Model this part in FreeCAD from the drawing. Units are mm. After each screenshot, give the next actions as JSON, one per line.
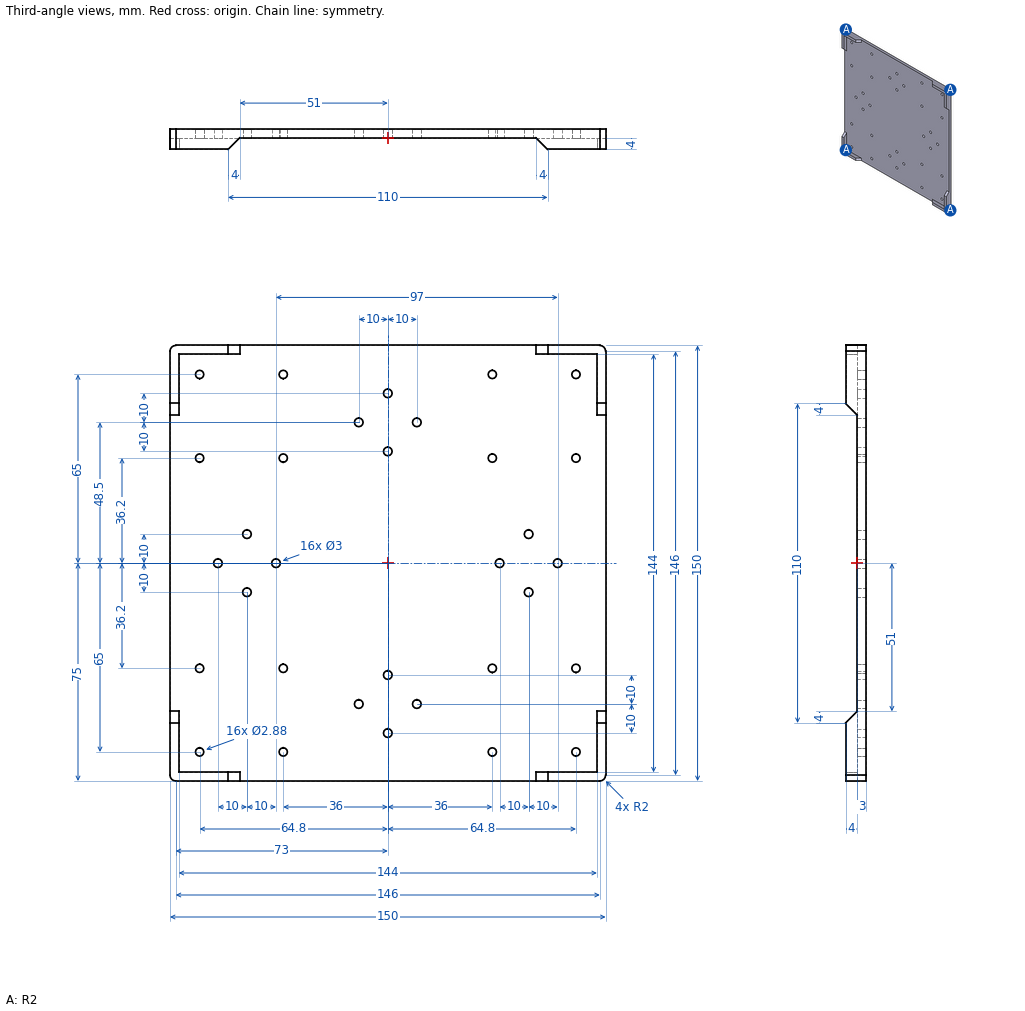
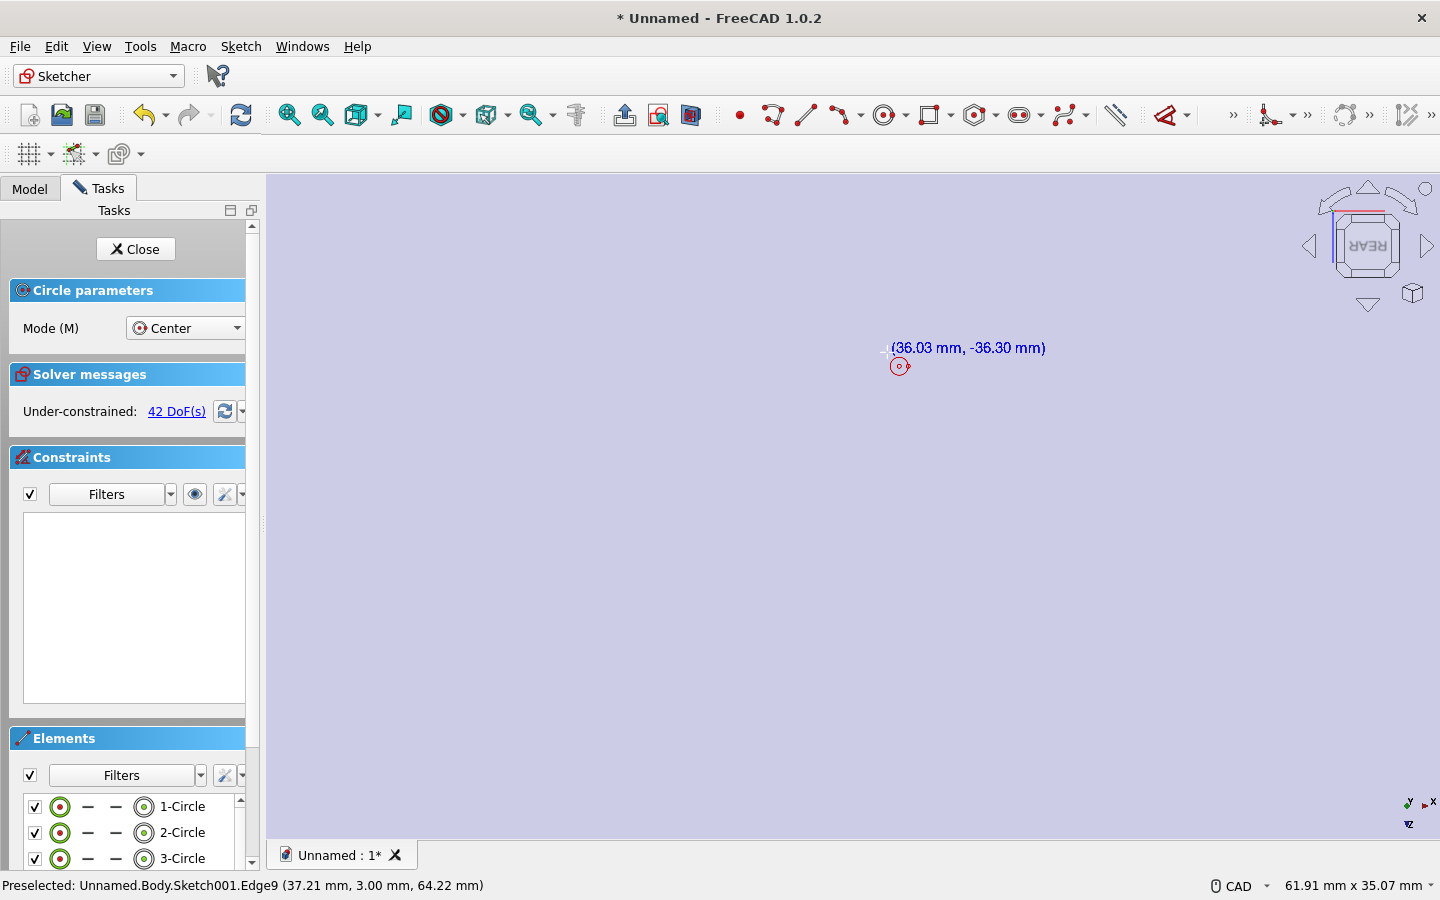
{"action": "scroll", "coordinate": [900, 673], "scroll_direction": "down", "scroll_amount": 9}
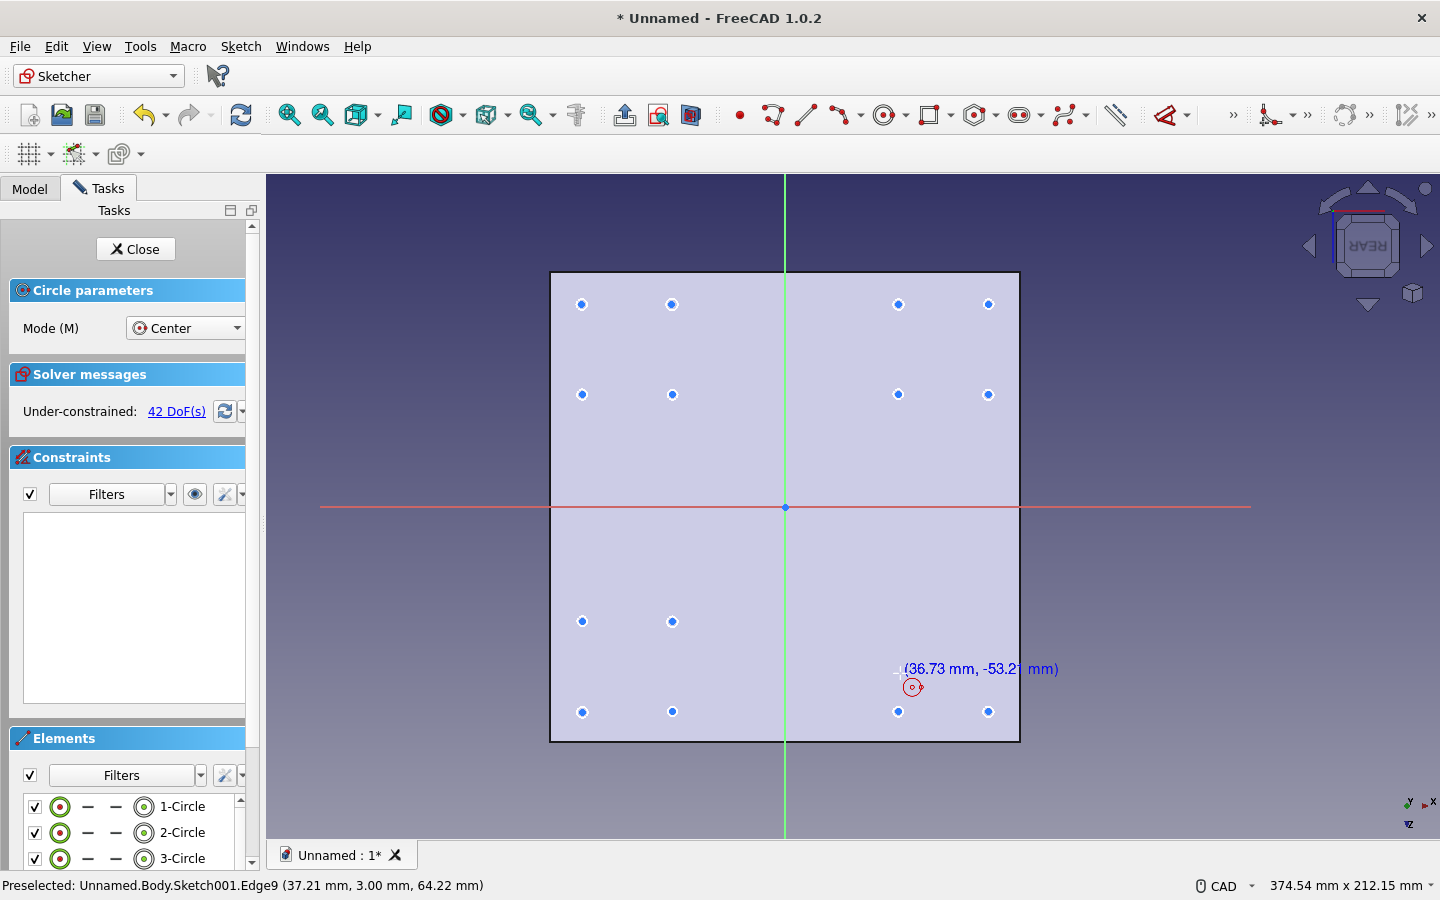
{"action": "left_click", "coordinate": [898, 620]}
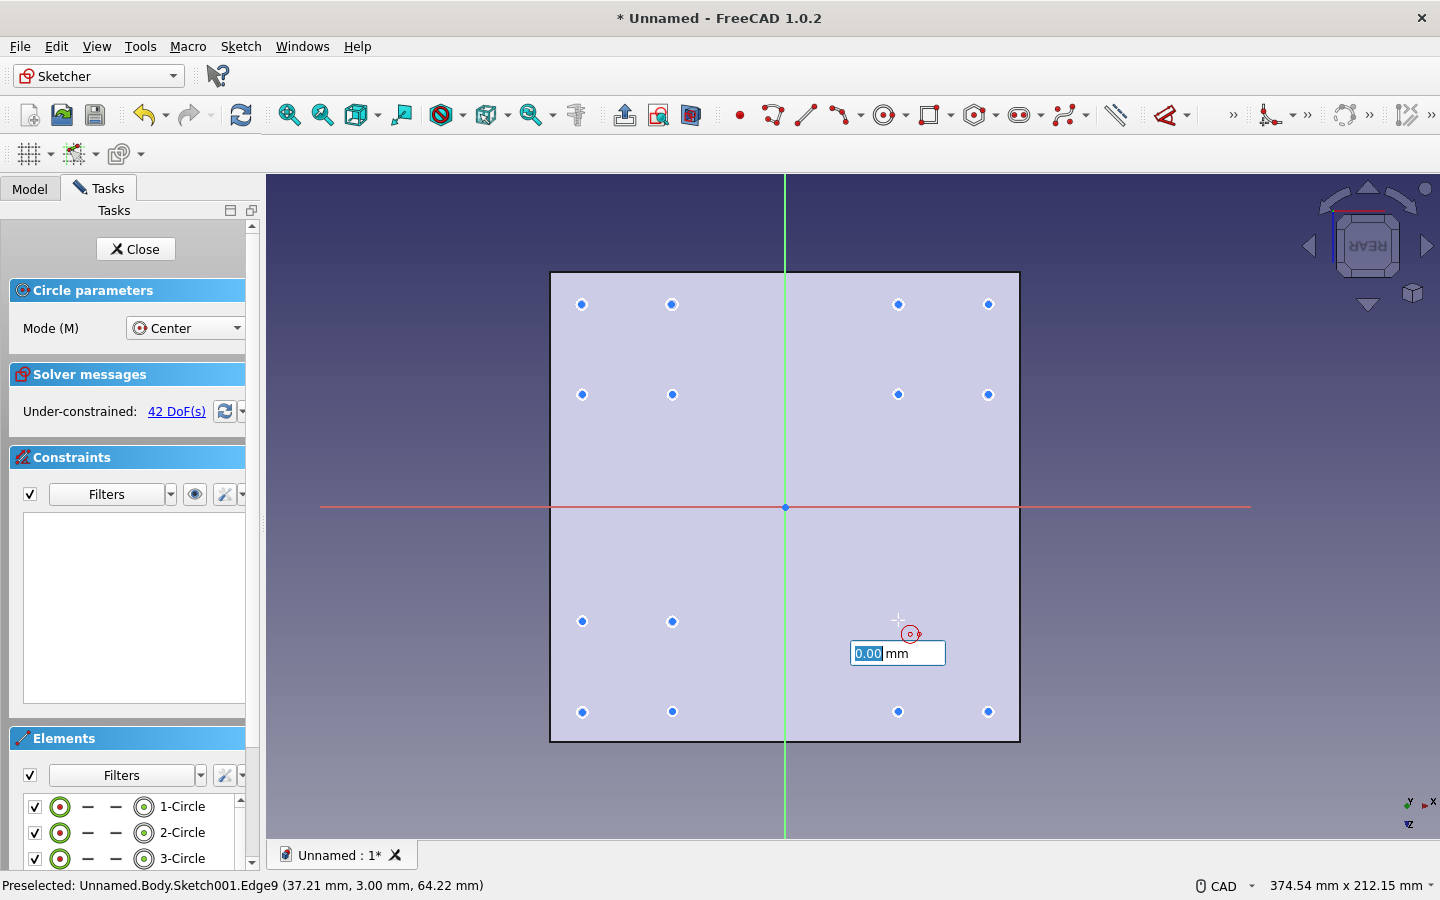
{"action": "scroll", "coordinate": [901, 617], "scroll_direction": "up", "scroll_amount": 7}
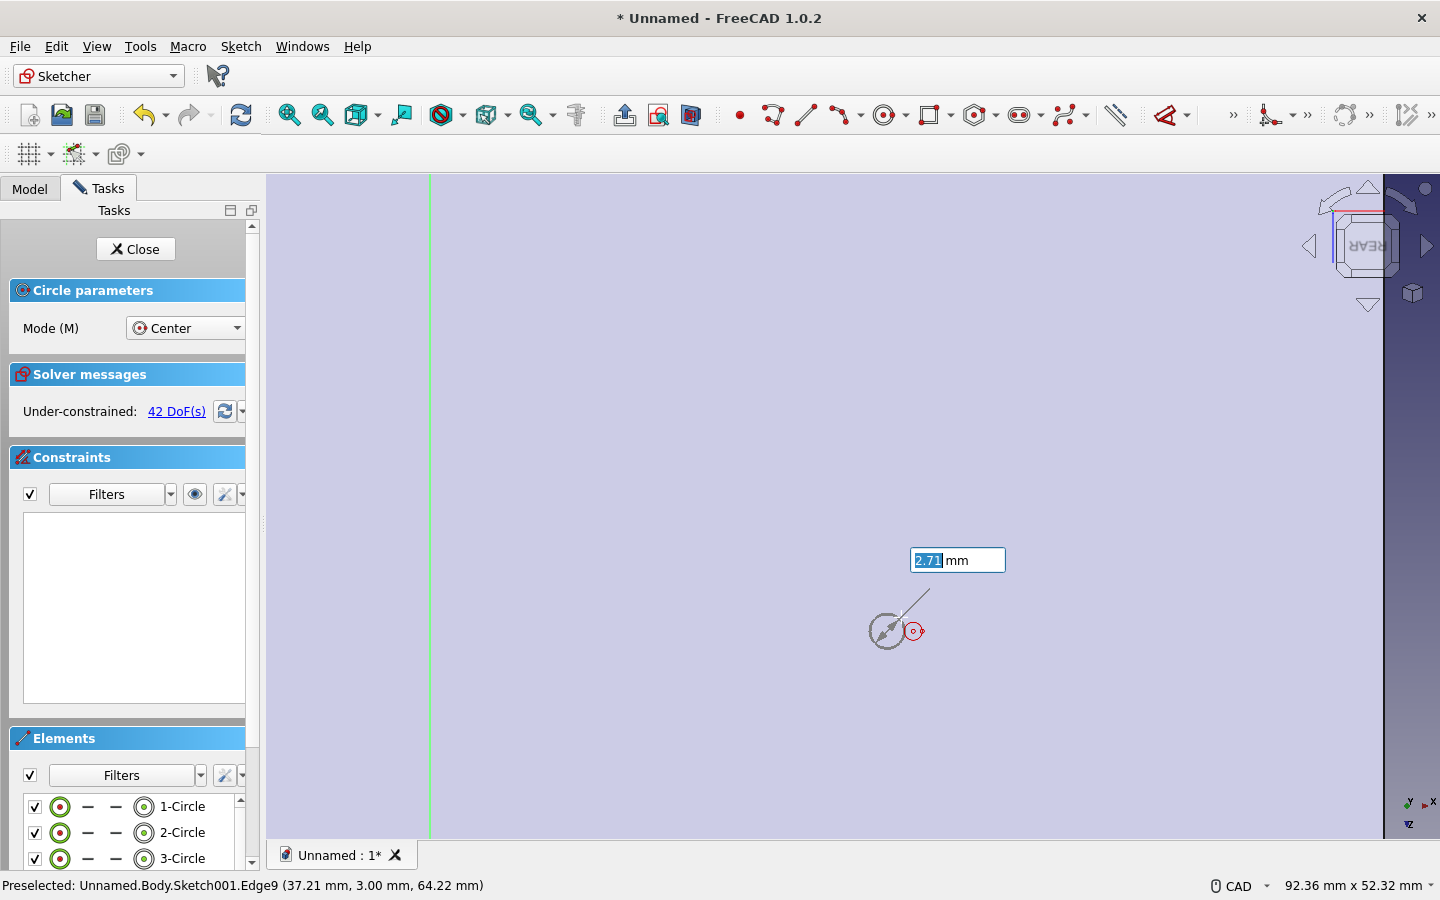
{"action": "left_click", "coordinate": [901, 616]}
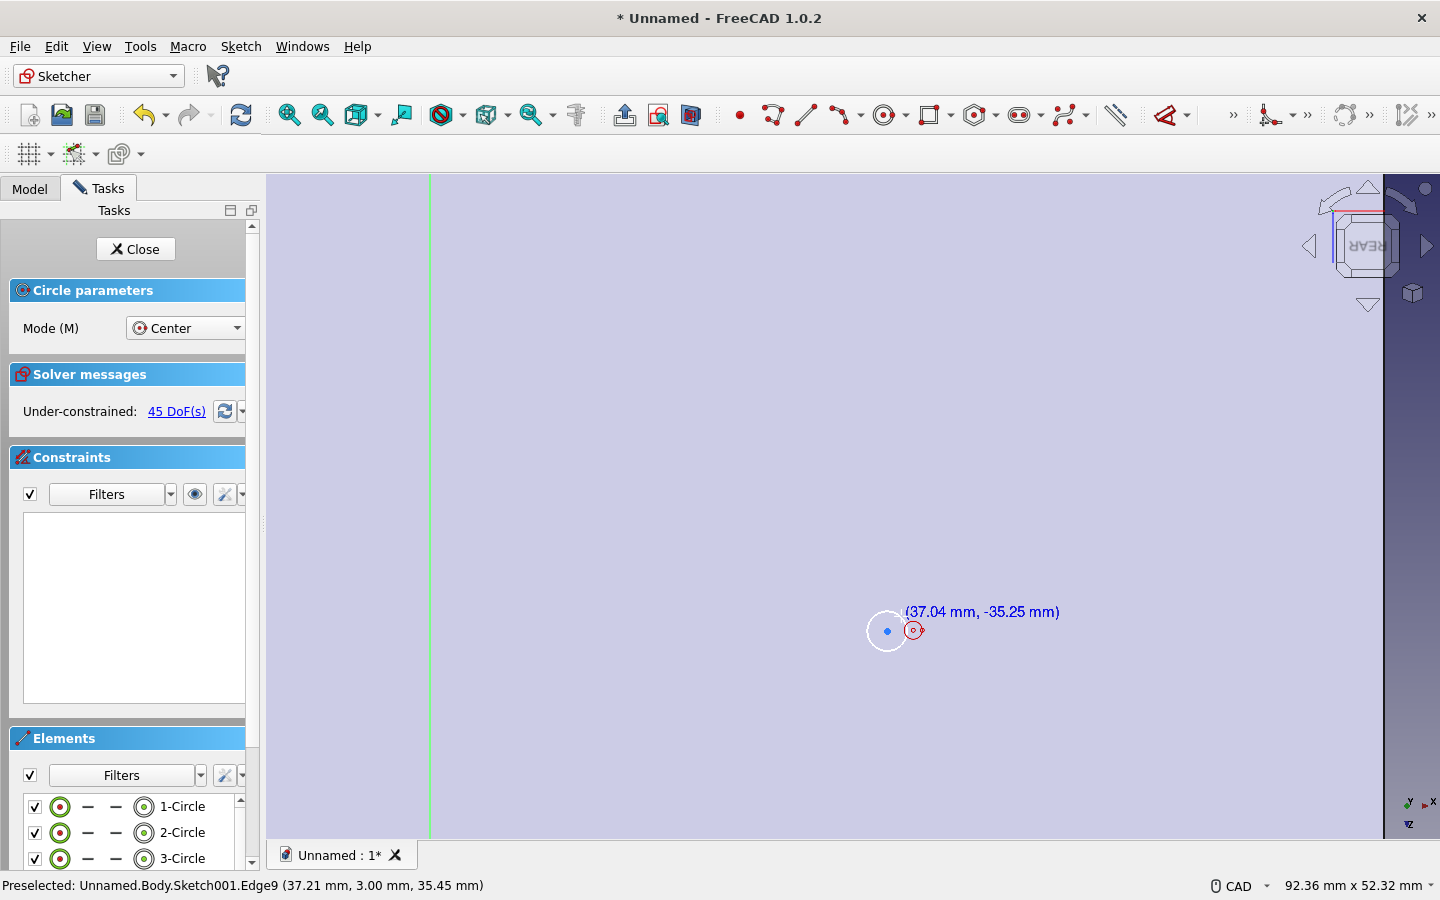
{"action": "scroll", "coordinate": [1254, 629], "scroll_direction": "up", "scroll_amount": 2}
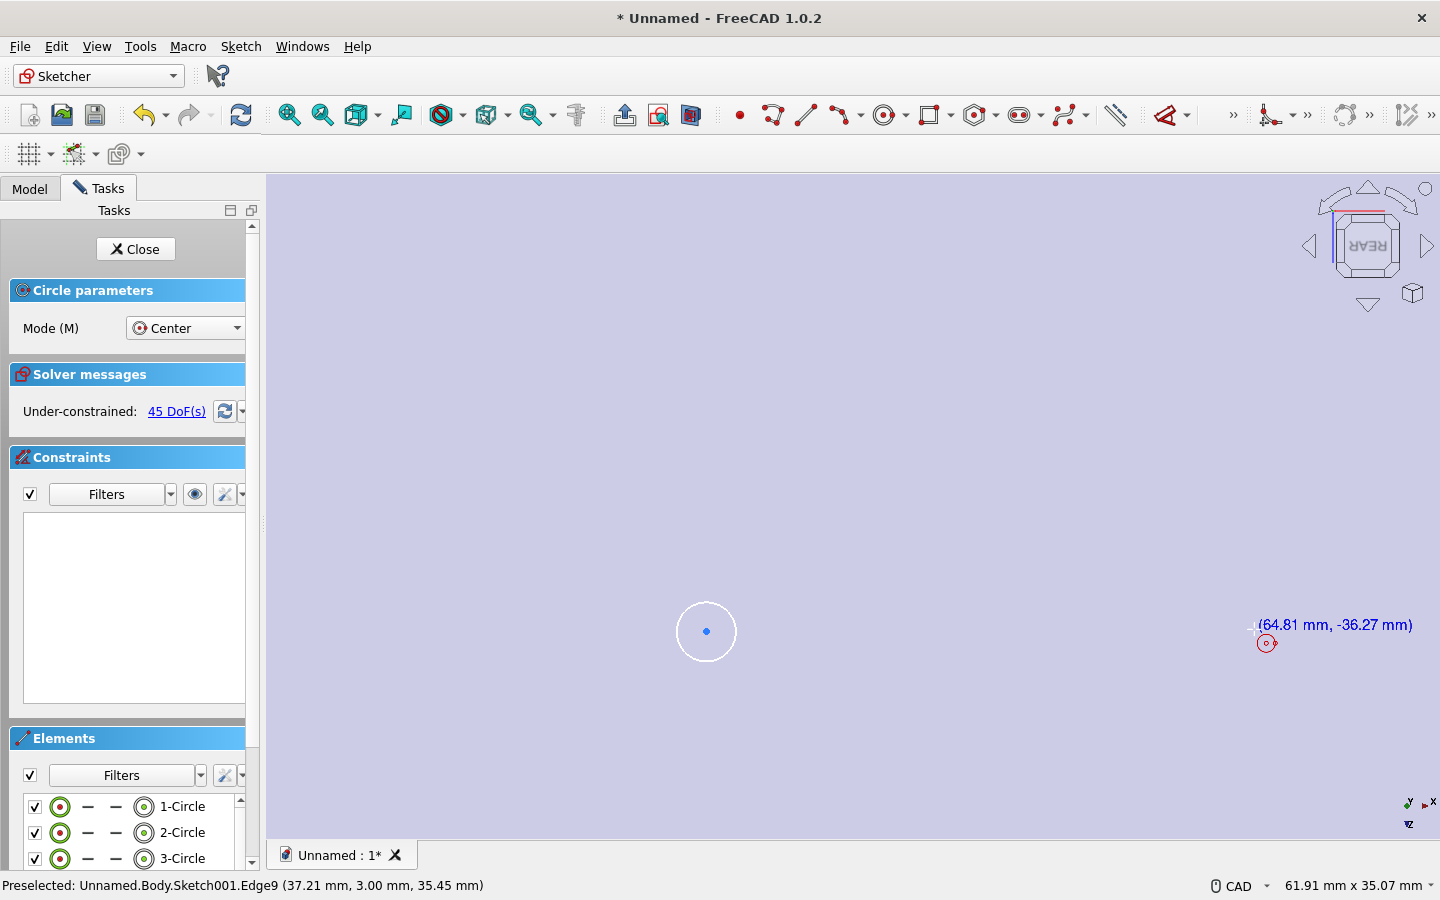
{"action": "scroll", "coordinate": [935, 618], "scroll_direction": "down", "scroll_amount": 9}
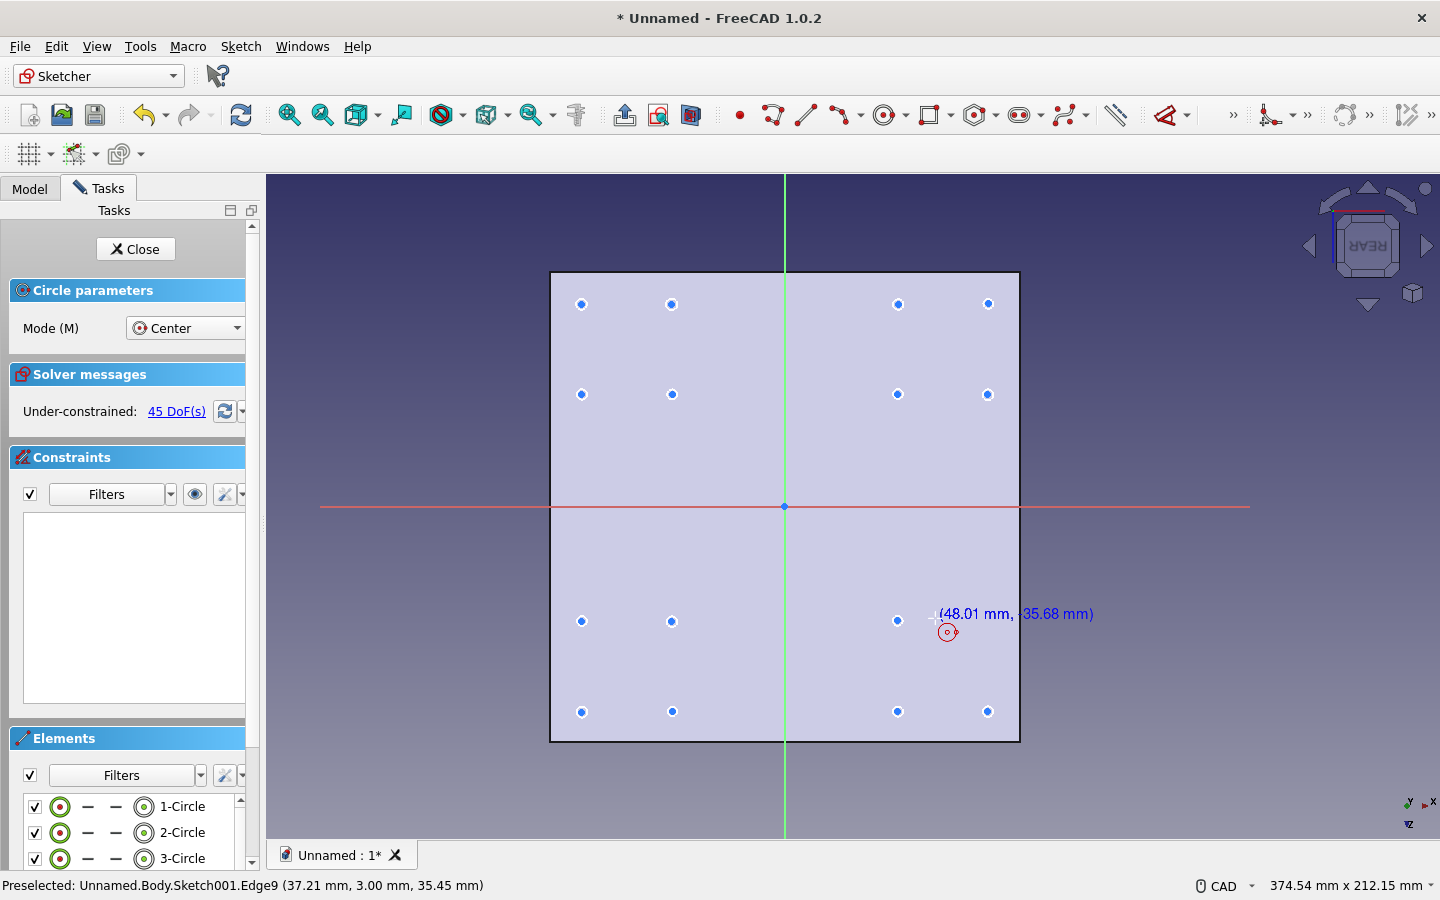
{"action": "left_click", "coordinate": [988, 620]}